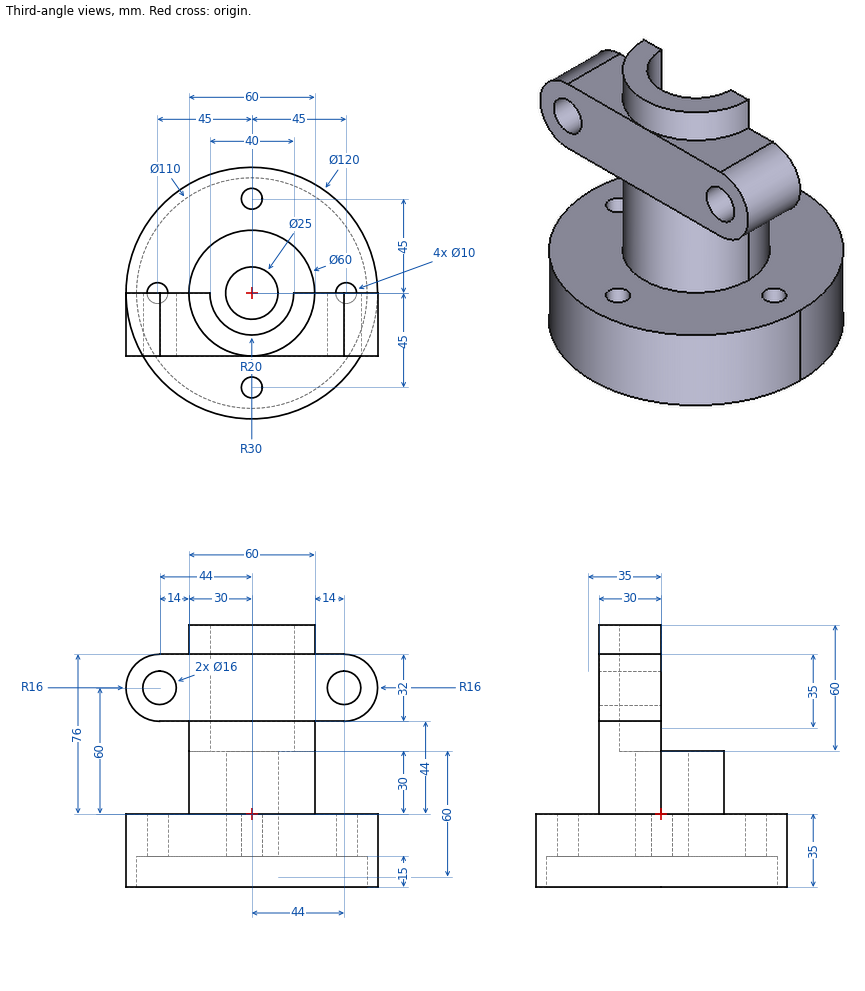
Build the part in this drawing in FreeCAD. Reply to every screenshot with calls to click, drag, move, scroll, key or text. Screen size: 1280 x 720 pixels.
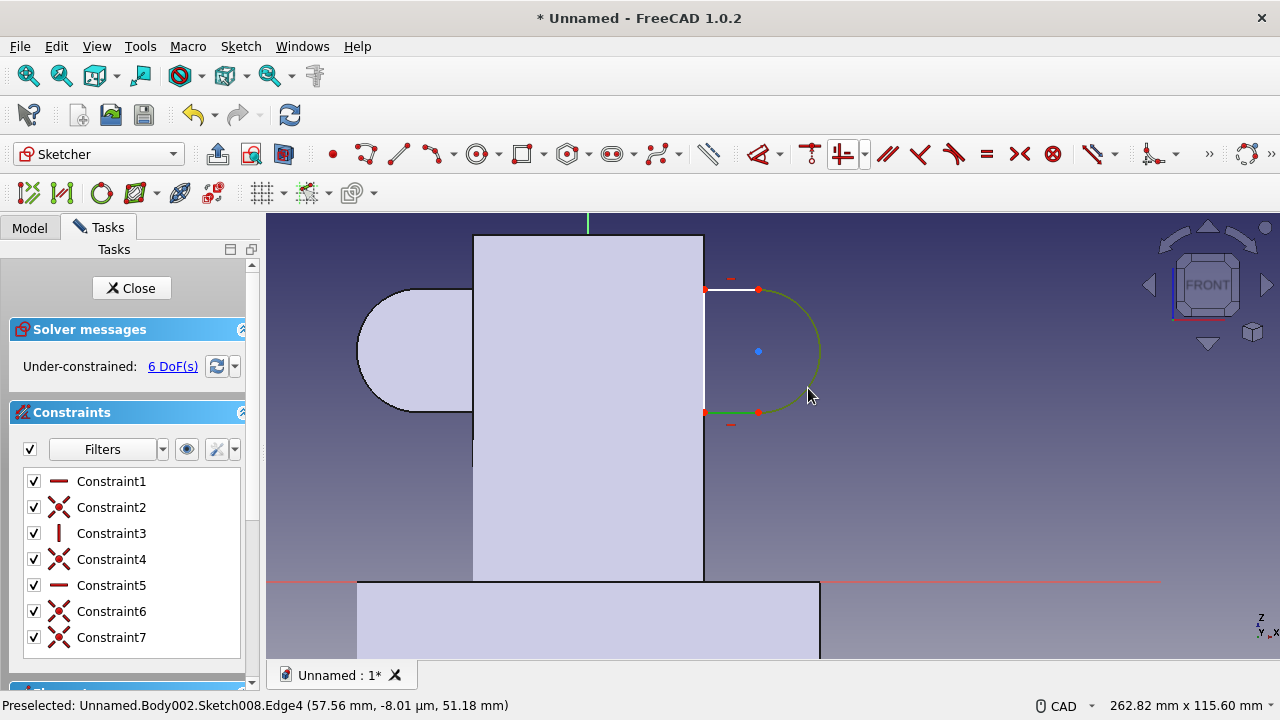
click(954, 154)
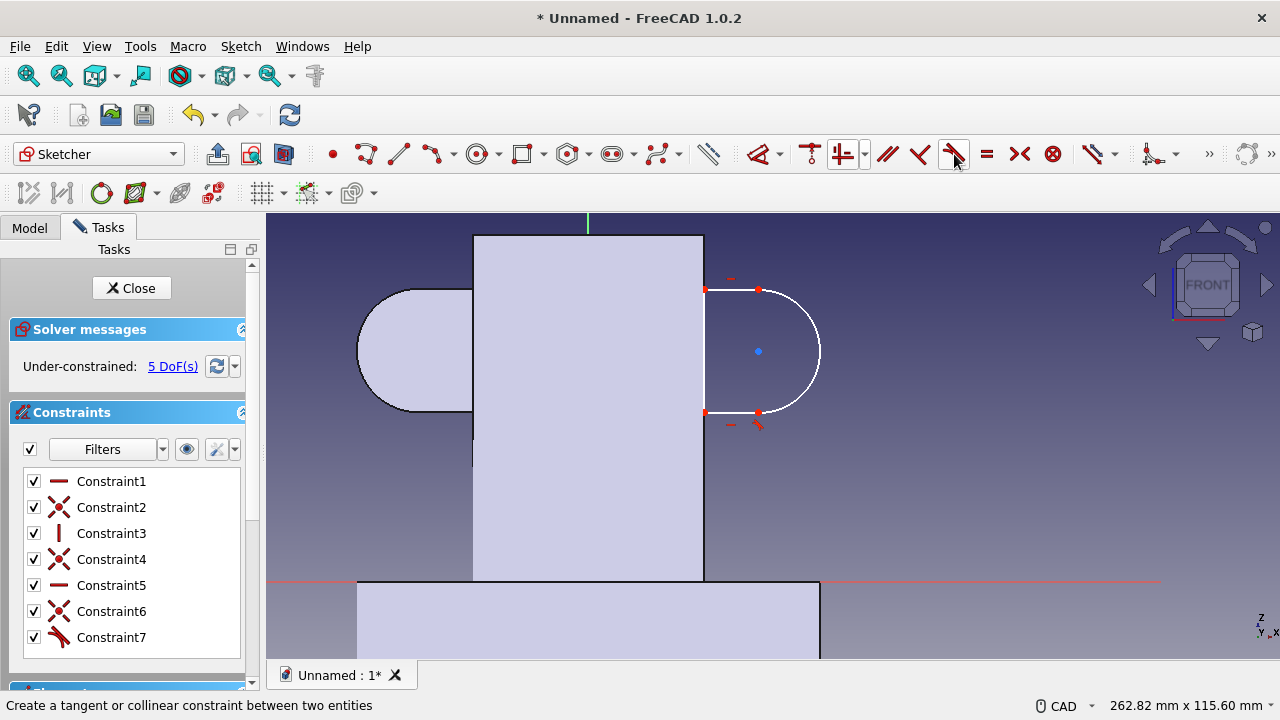
click(720, 290)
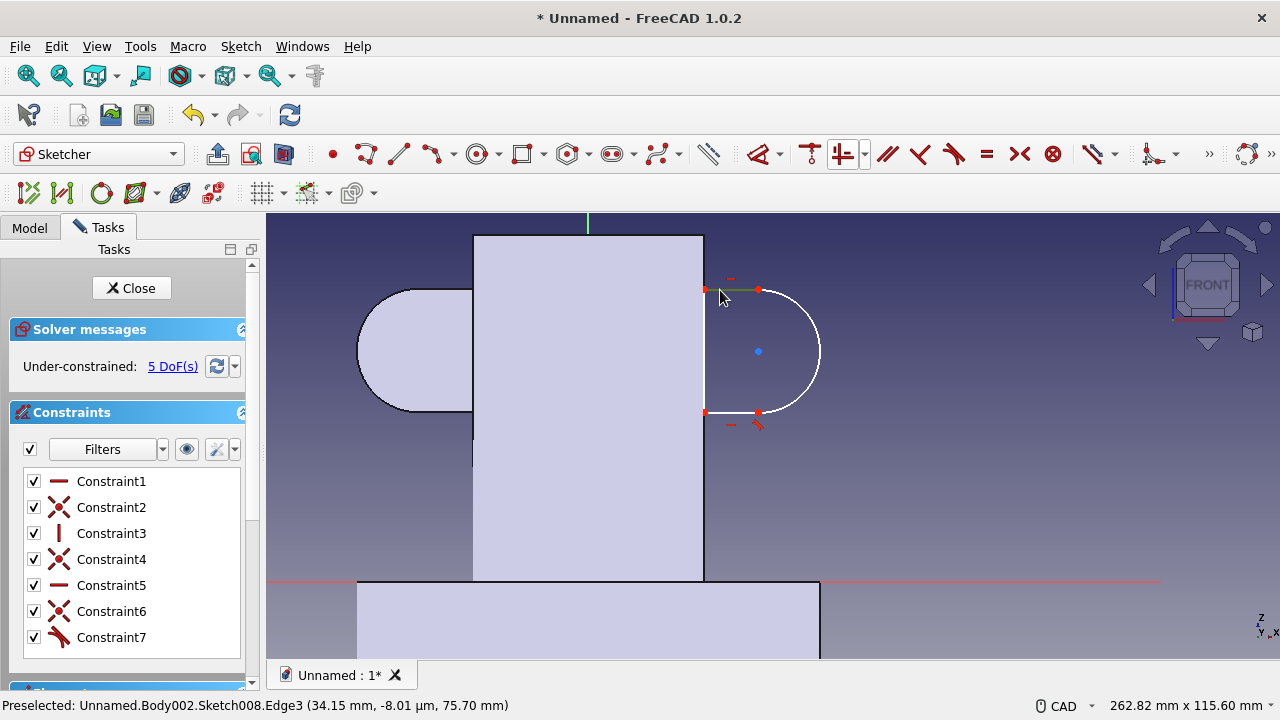
click(808, 388)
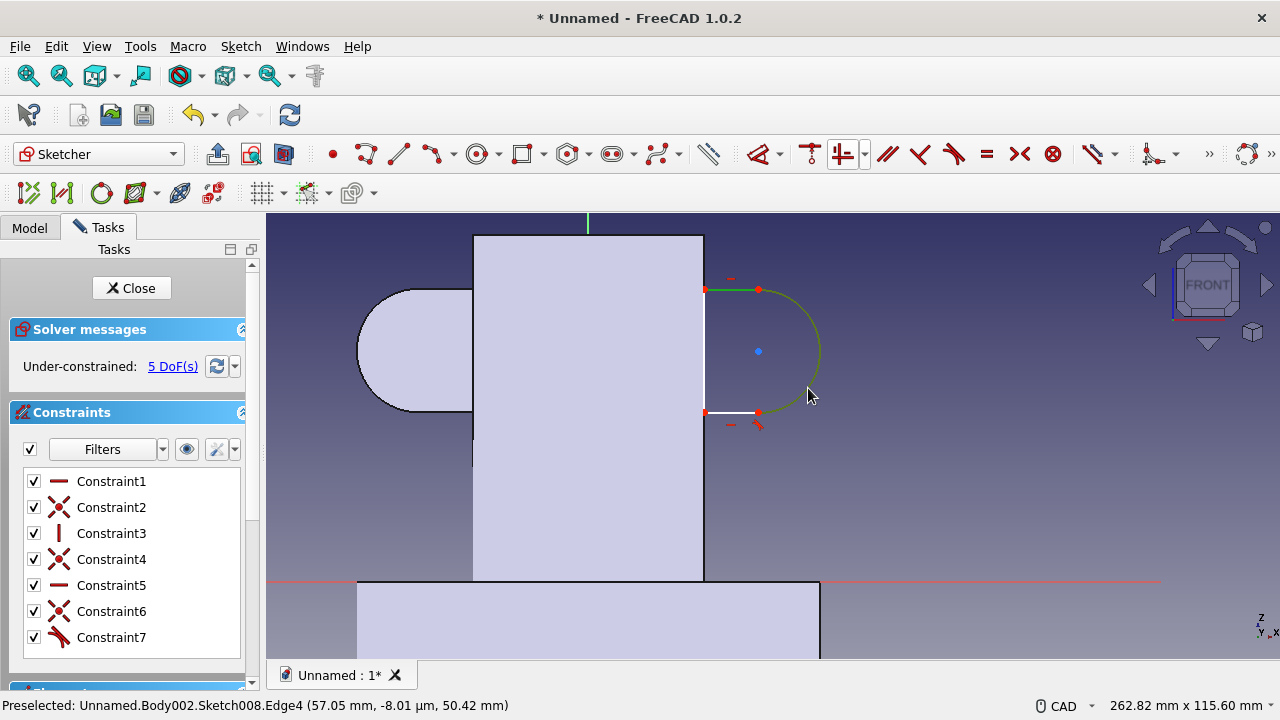
click(954, 154)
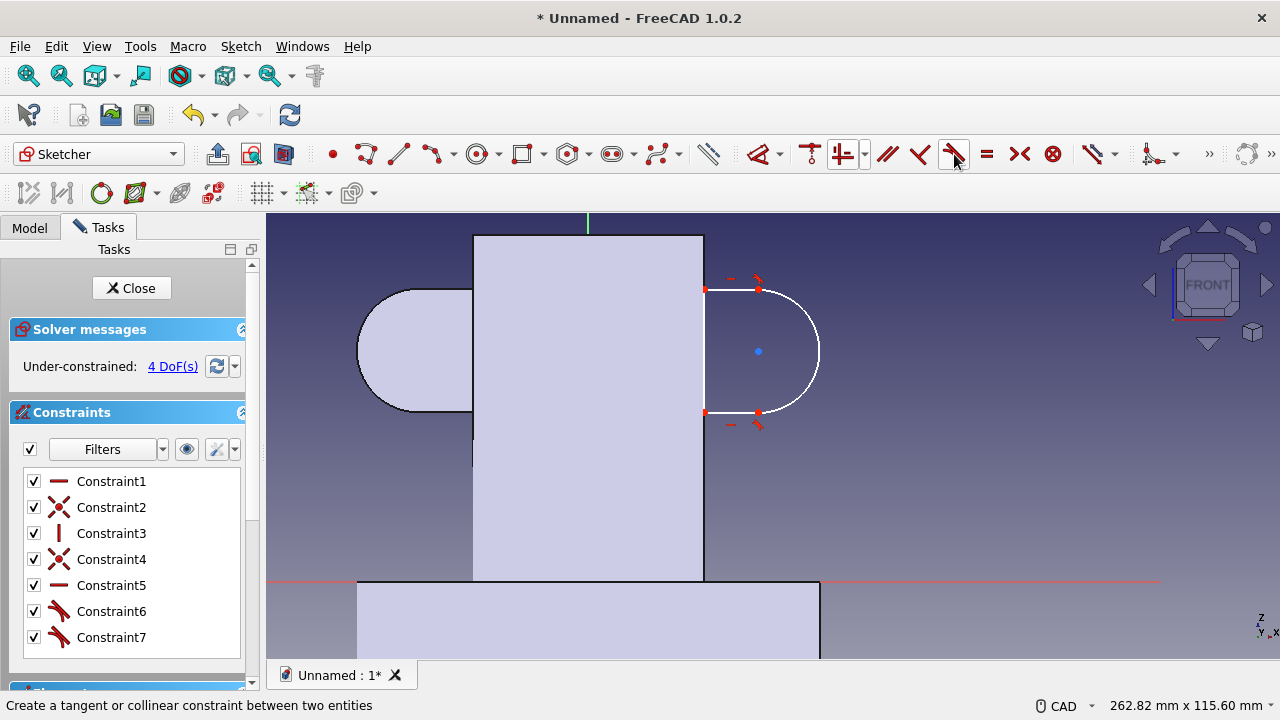
click(758, 154)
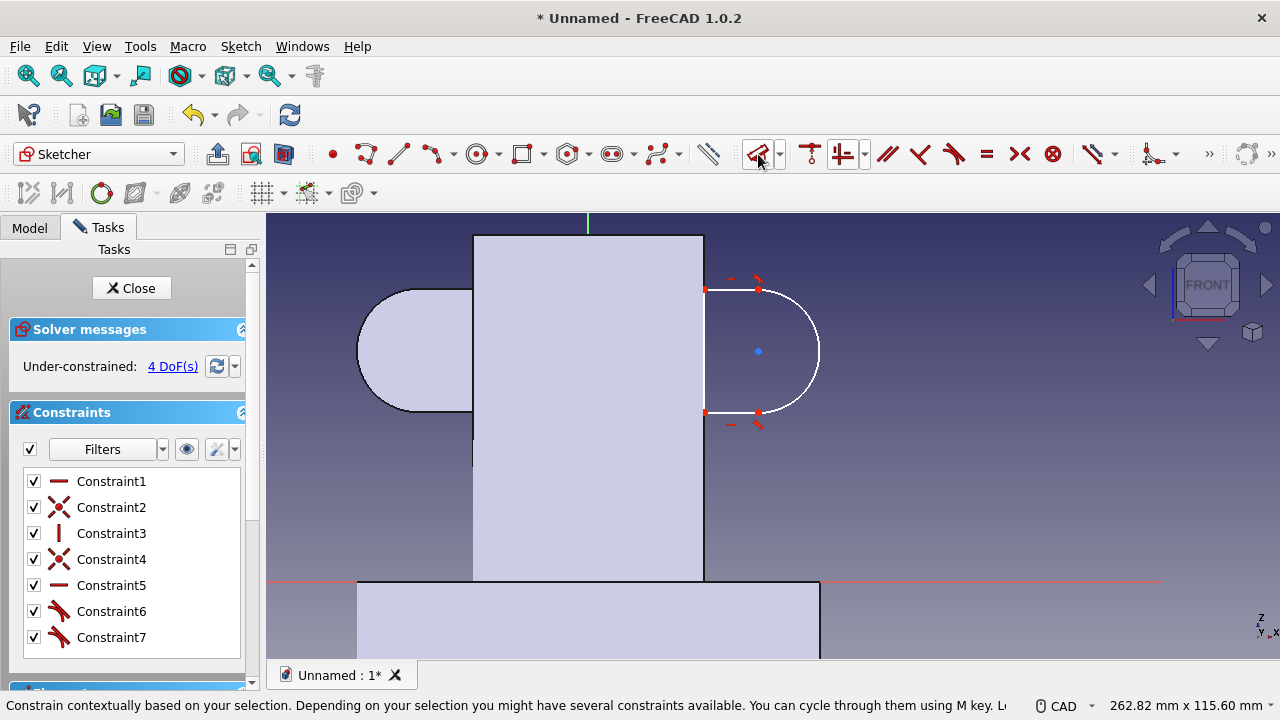
click(808, 388)
click(834, 407)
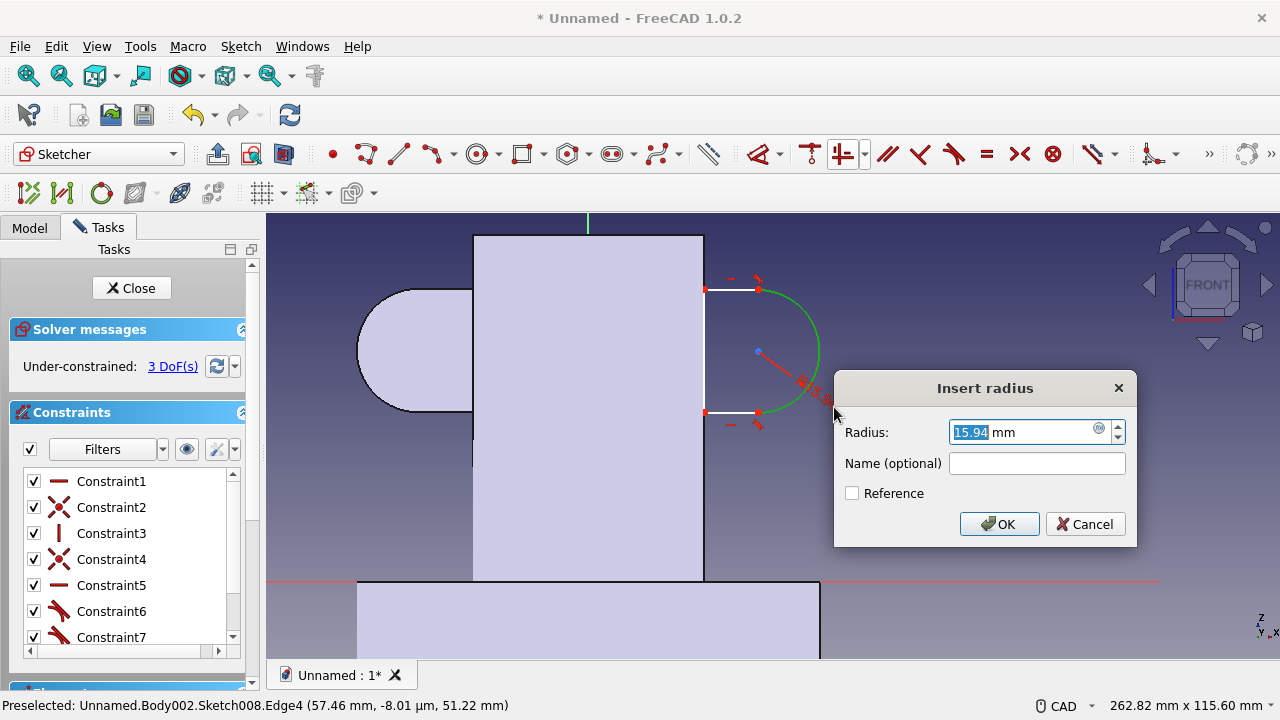
text(16)
key(Return)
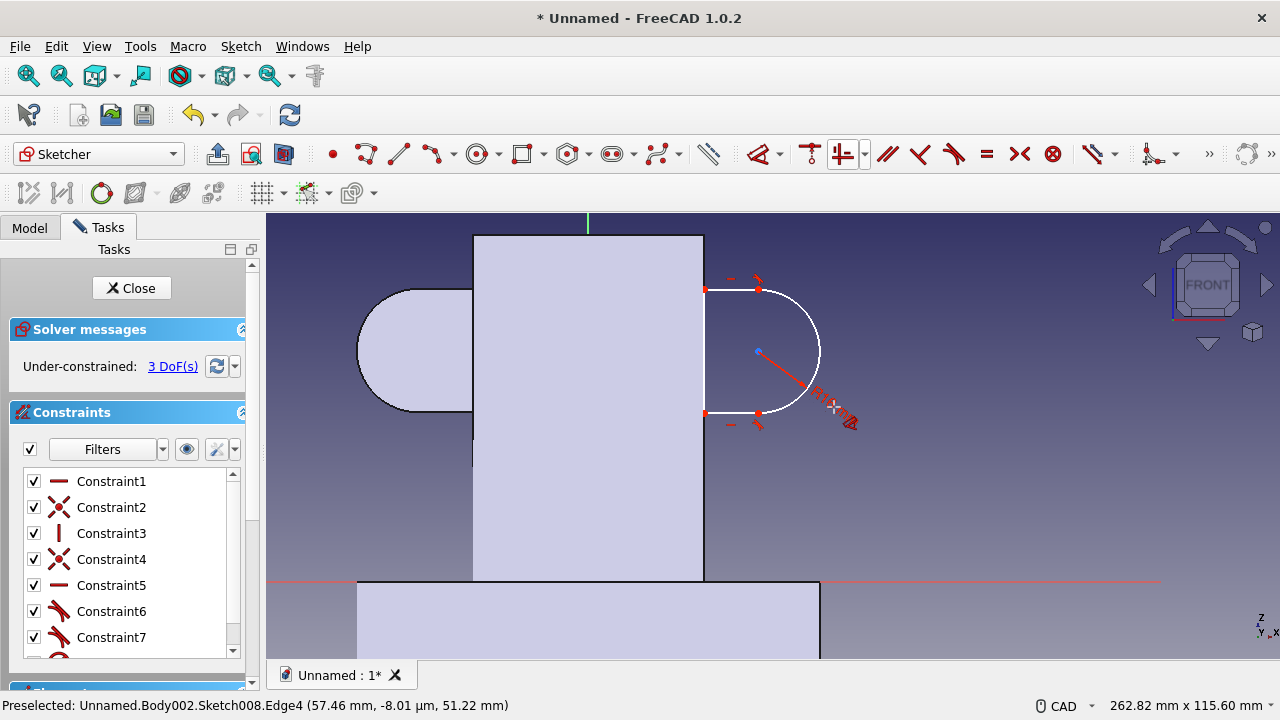
click(742, 413)
click(731, 379)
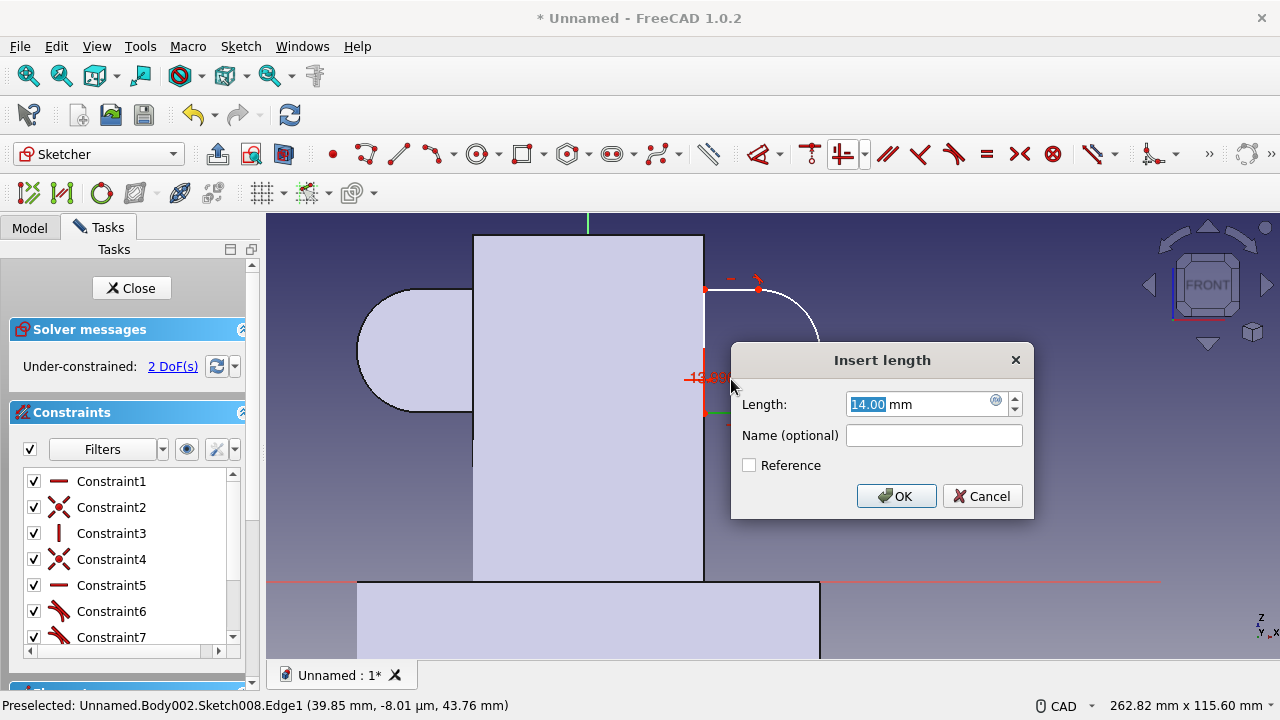
text(14)
key(Return)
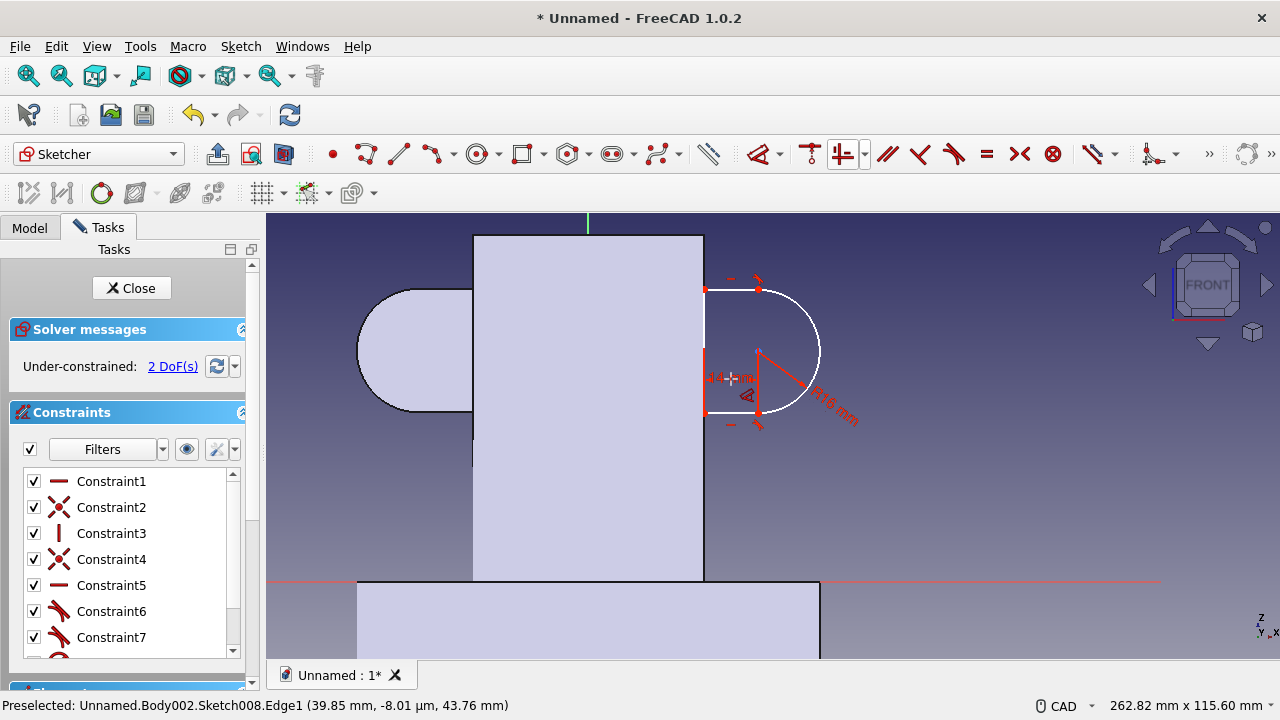
click(758, 413)
click(673, 616)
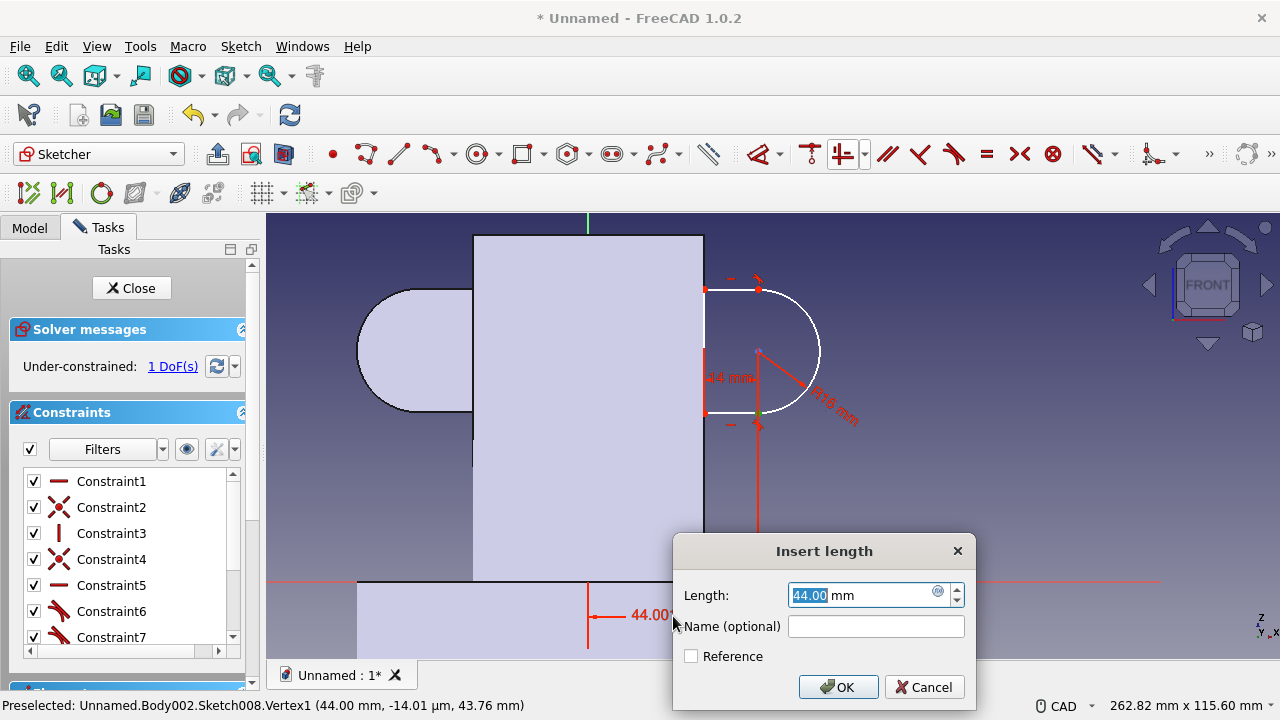
text(44)
key(Return)